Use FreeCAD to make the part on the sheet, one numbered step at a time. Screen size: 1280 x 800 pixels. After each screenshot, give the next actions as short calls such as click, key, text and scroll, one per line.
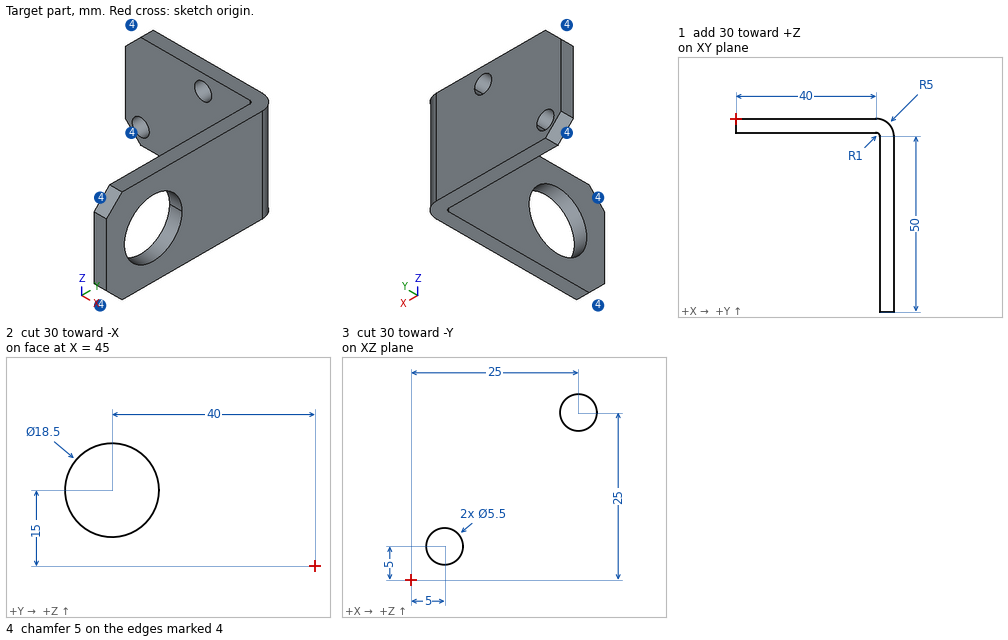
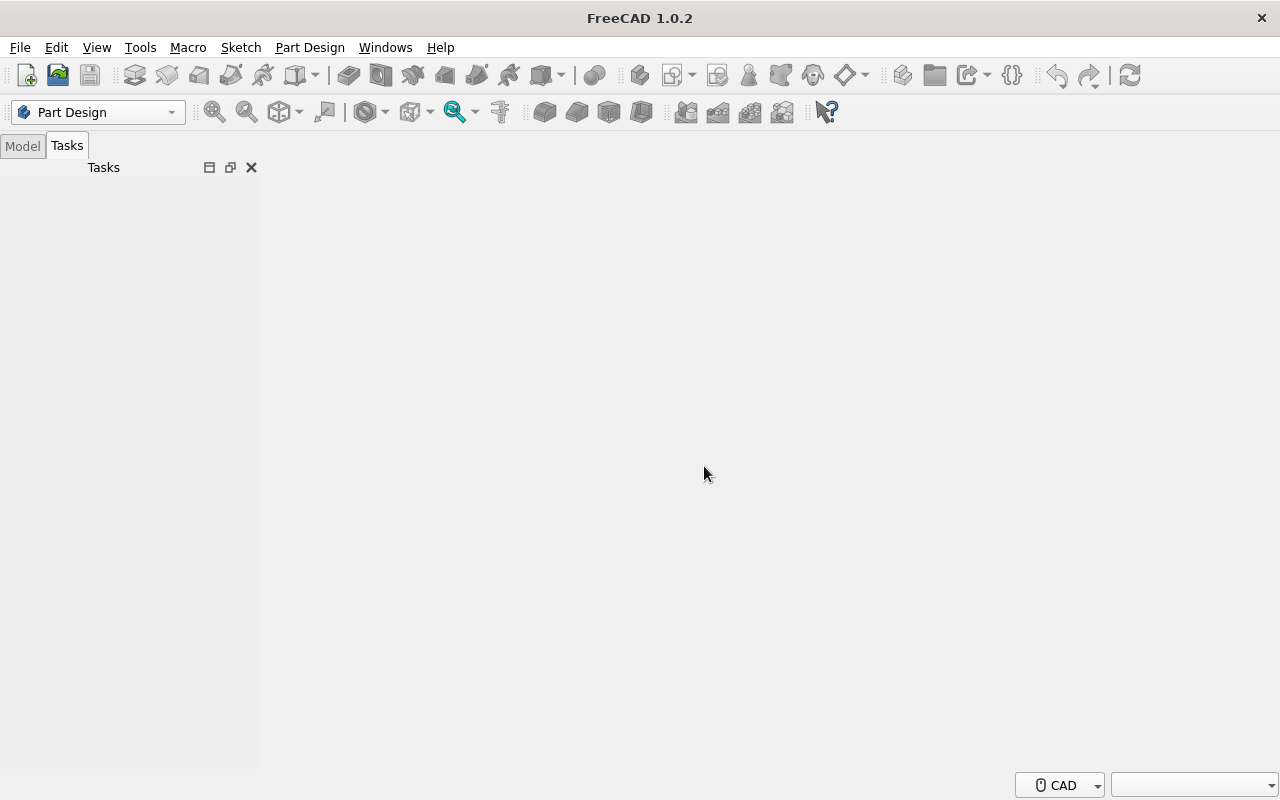
click(26, 76)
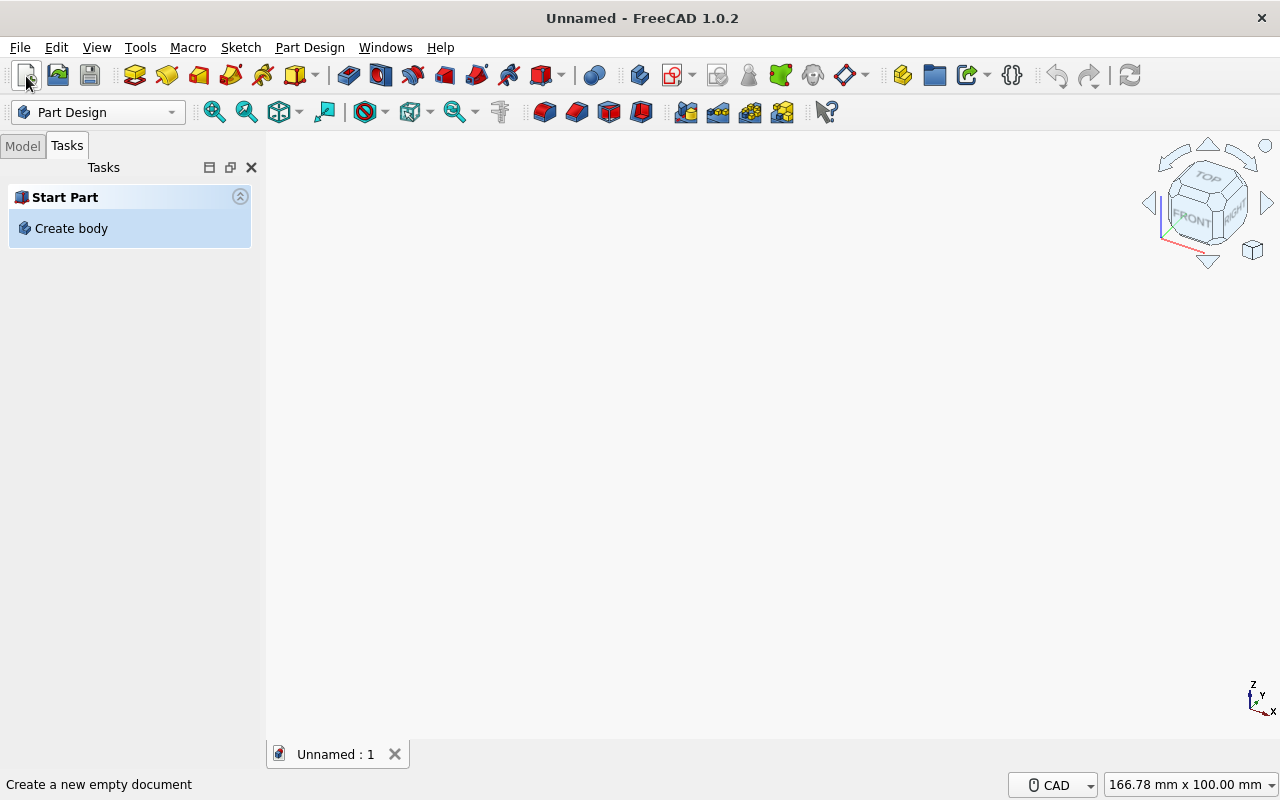
click(672, 76)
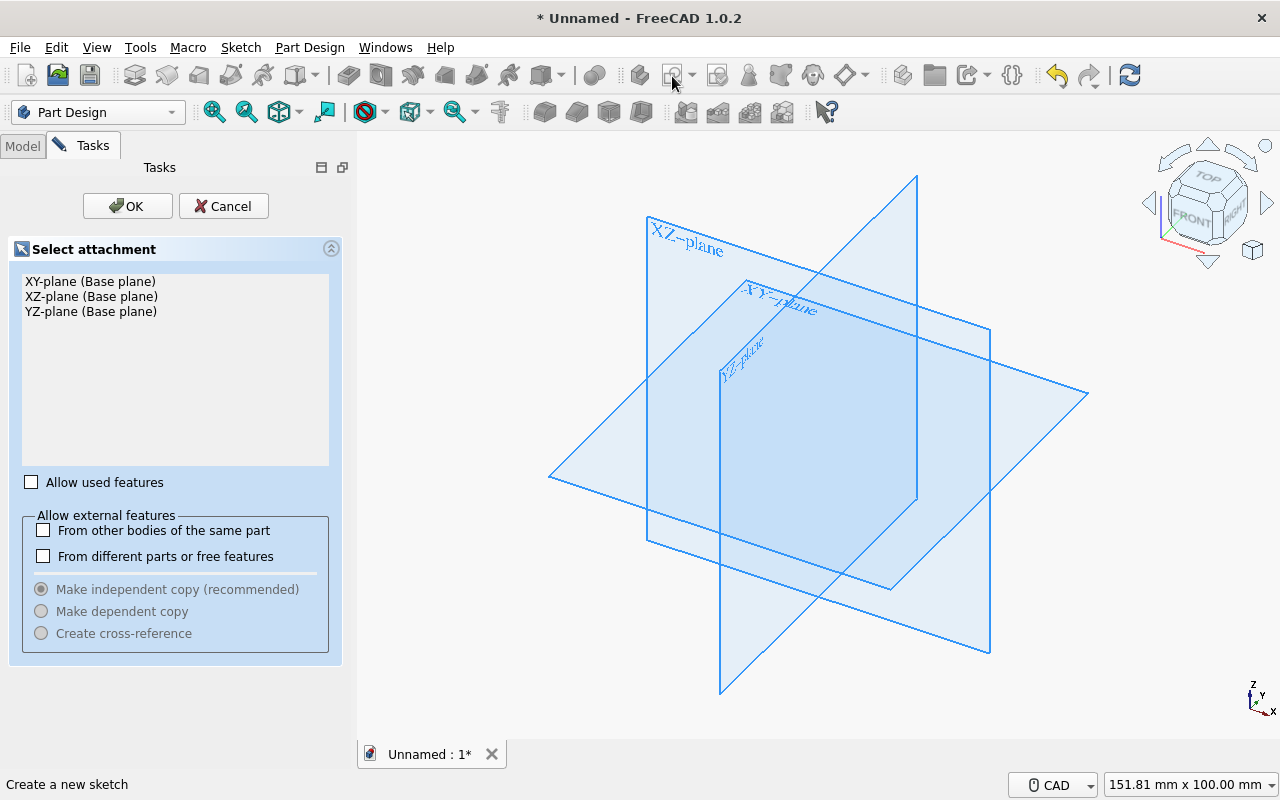
click(82, 282)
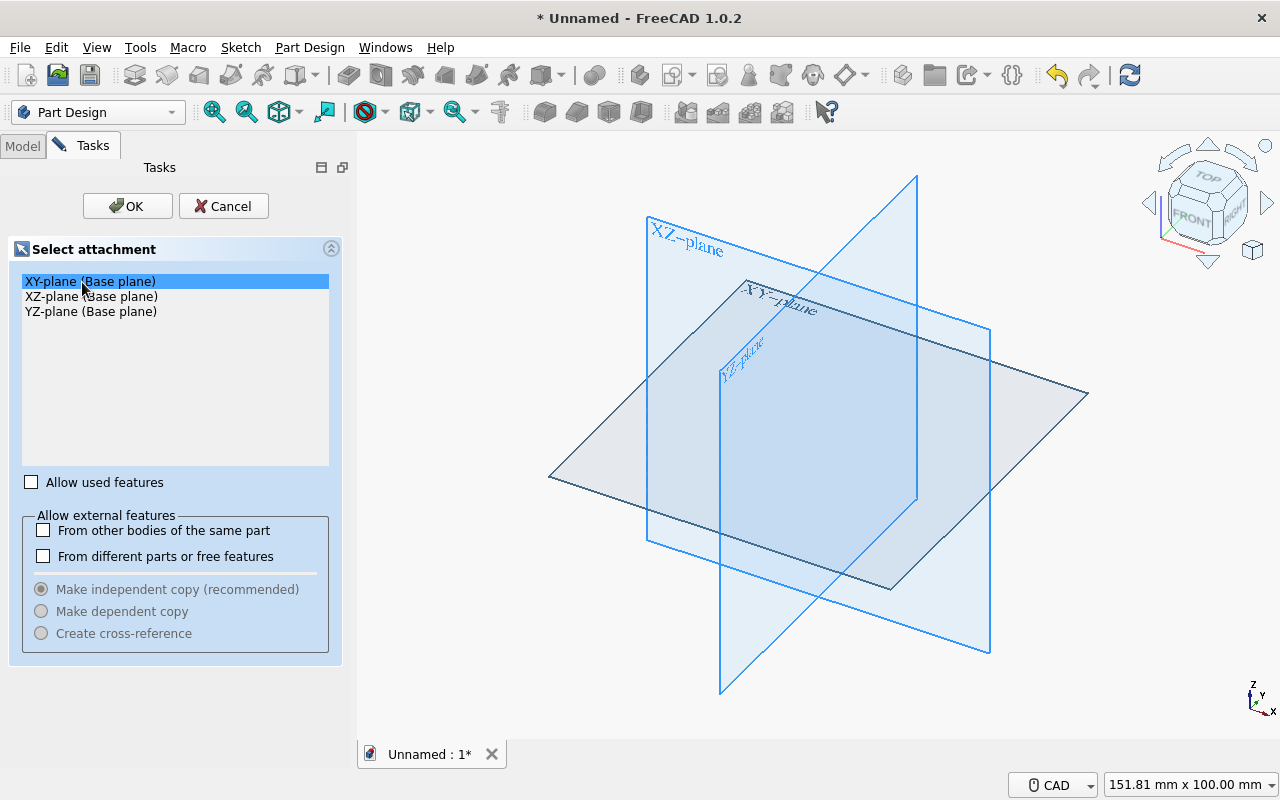
click(128, 206)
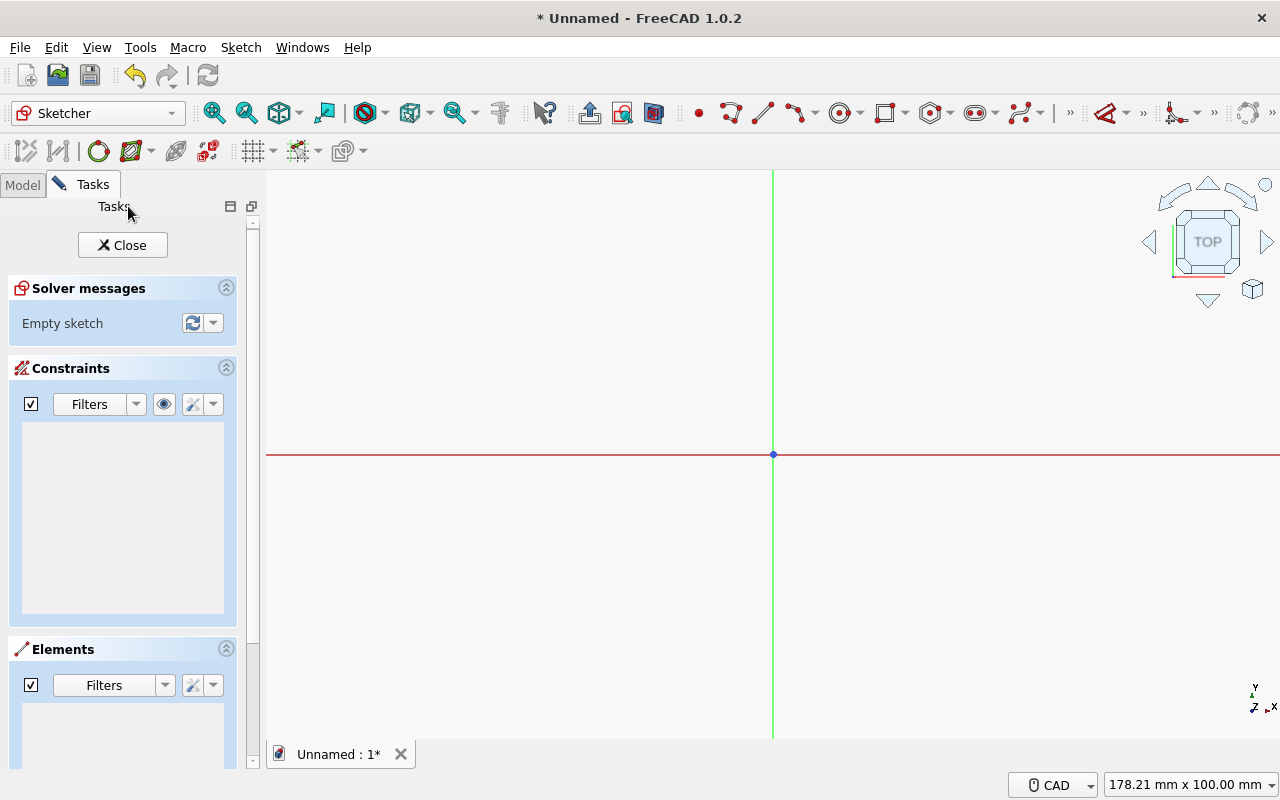
scroll(294, 198, down, 1)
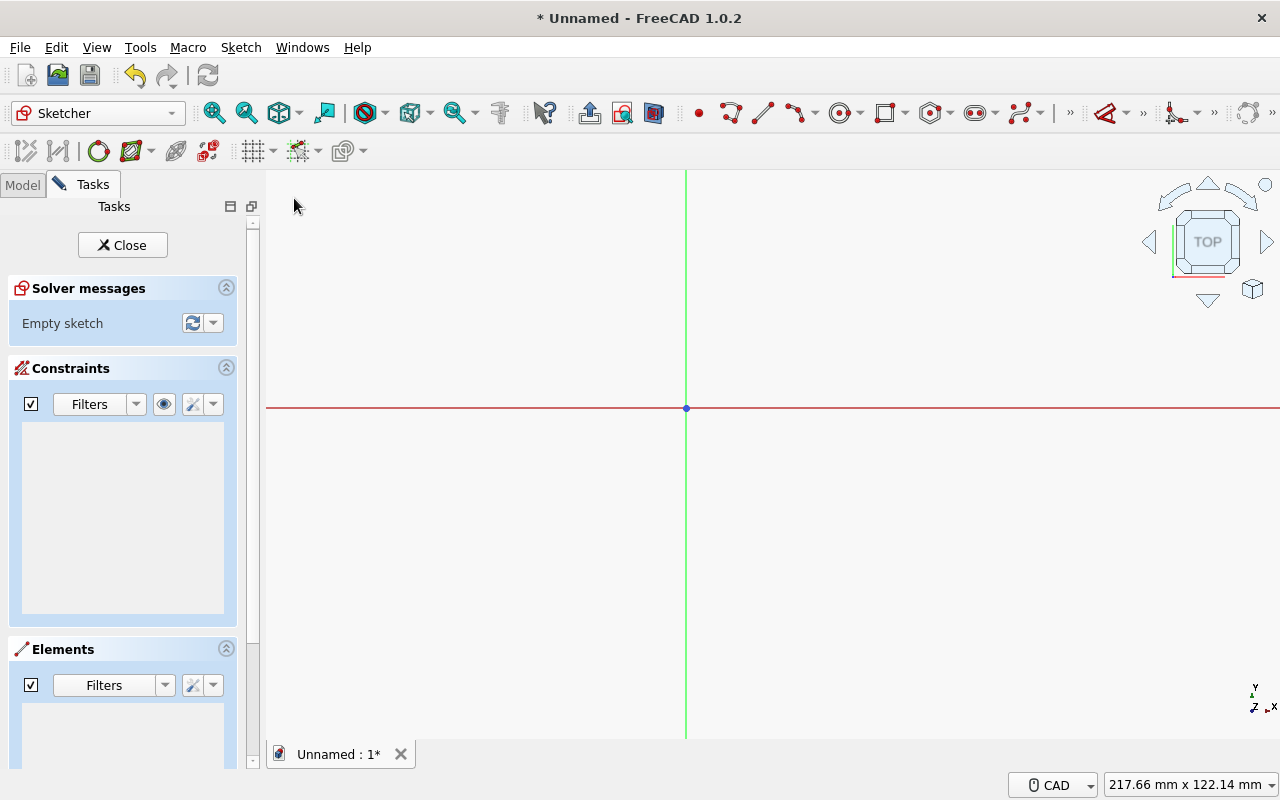
scroll(967, 702, up, 2)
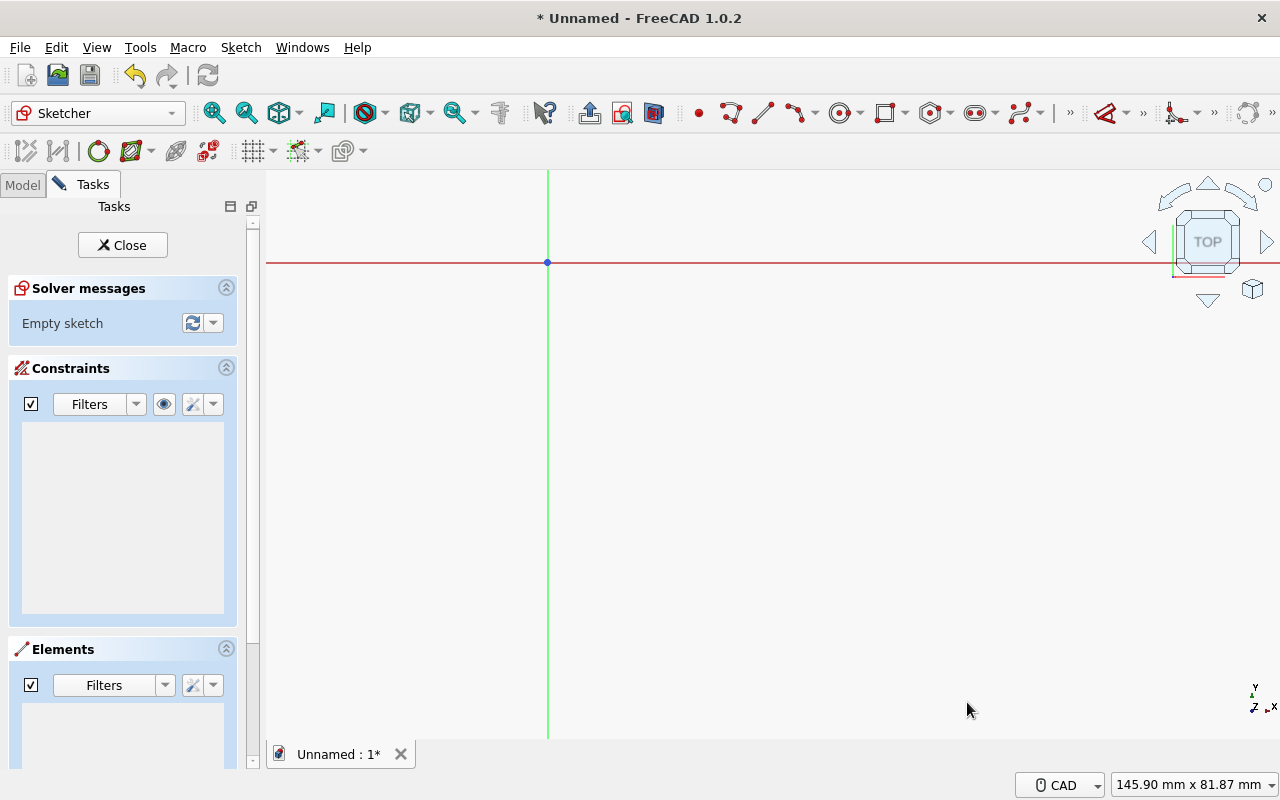
key(g)
key(m)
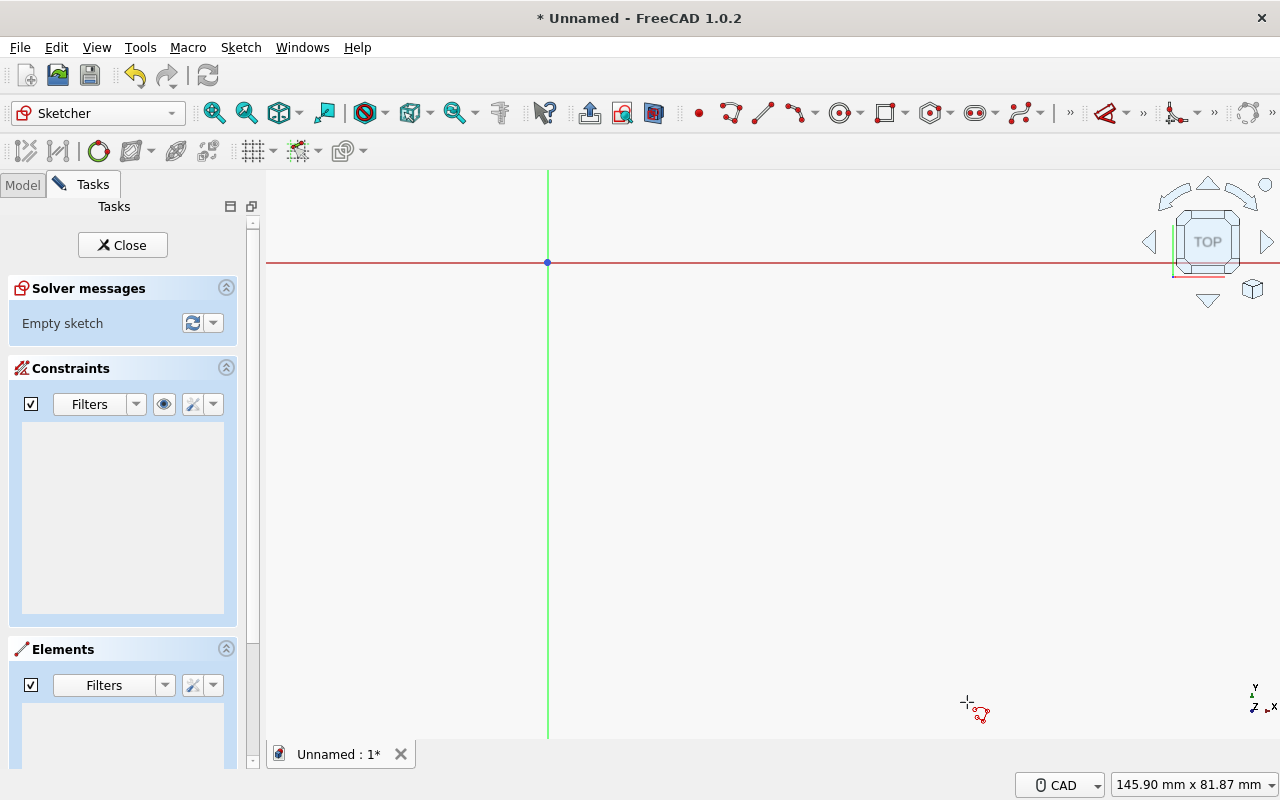
click(826, 263)
click(548, 263)
click(557, 291)
click(826, 291)
right_click(826, 291)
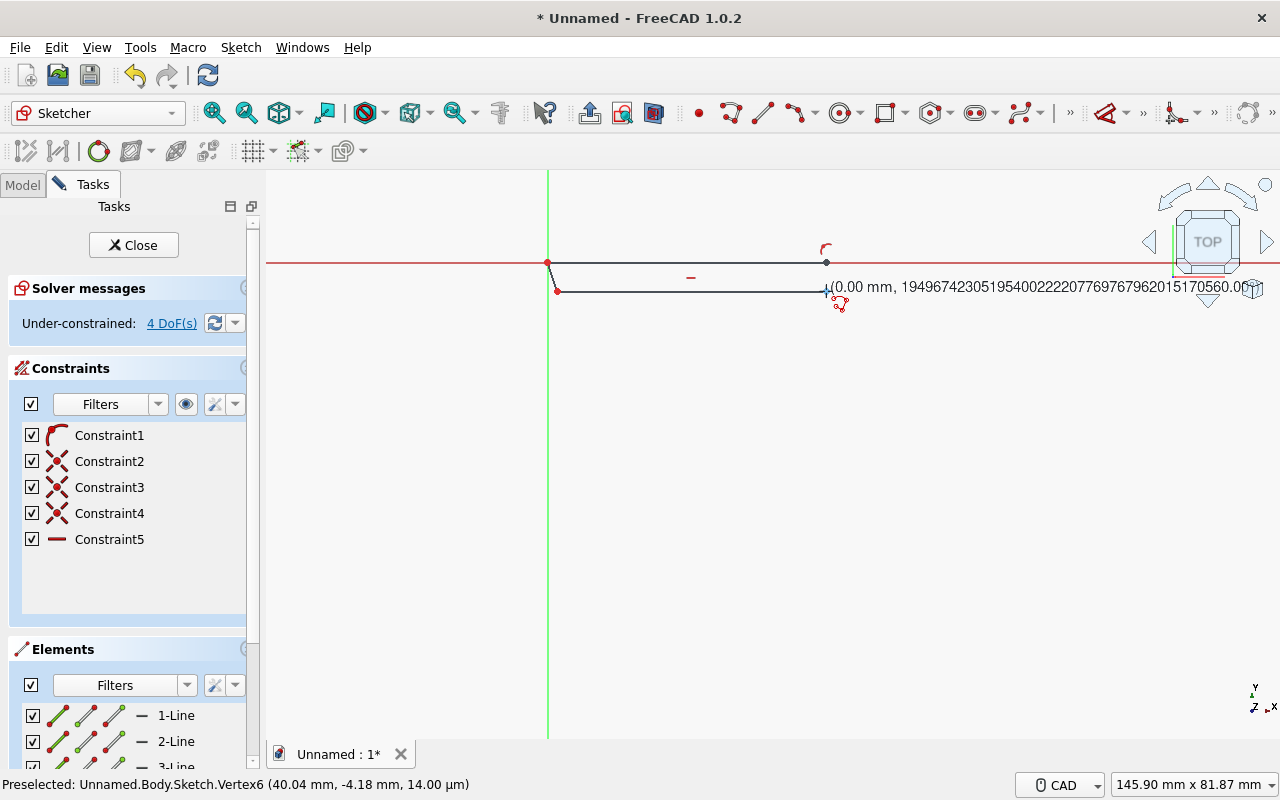
scroll(833, 298, up, 3)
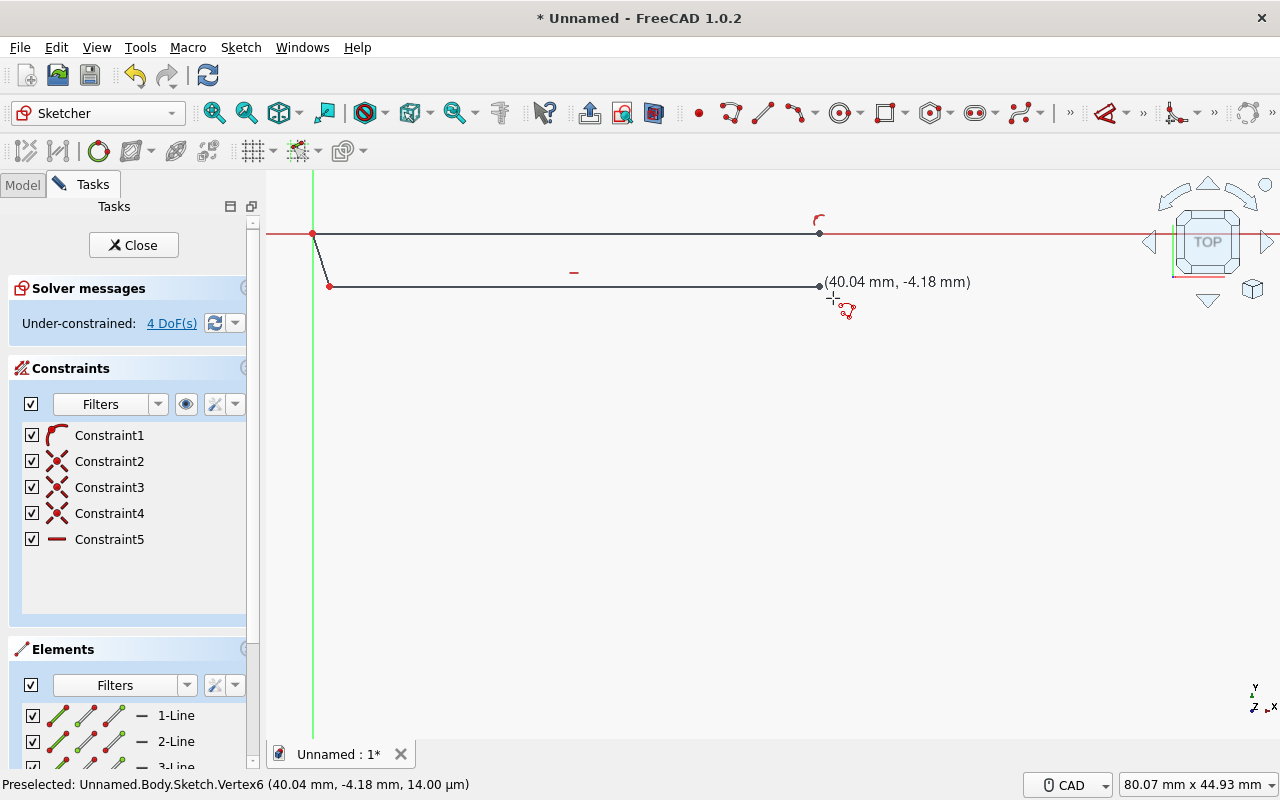
click(832, 297)